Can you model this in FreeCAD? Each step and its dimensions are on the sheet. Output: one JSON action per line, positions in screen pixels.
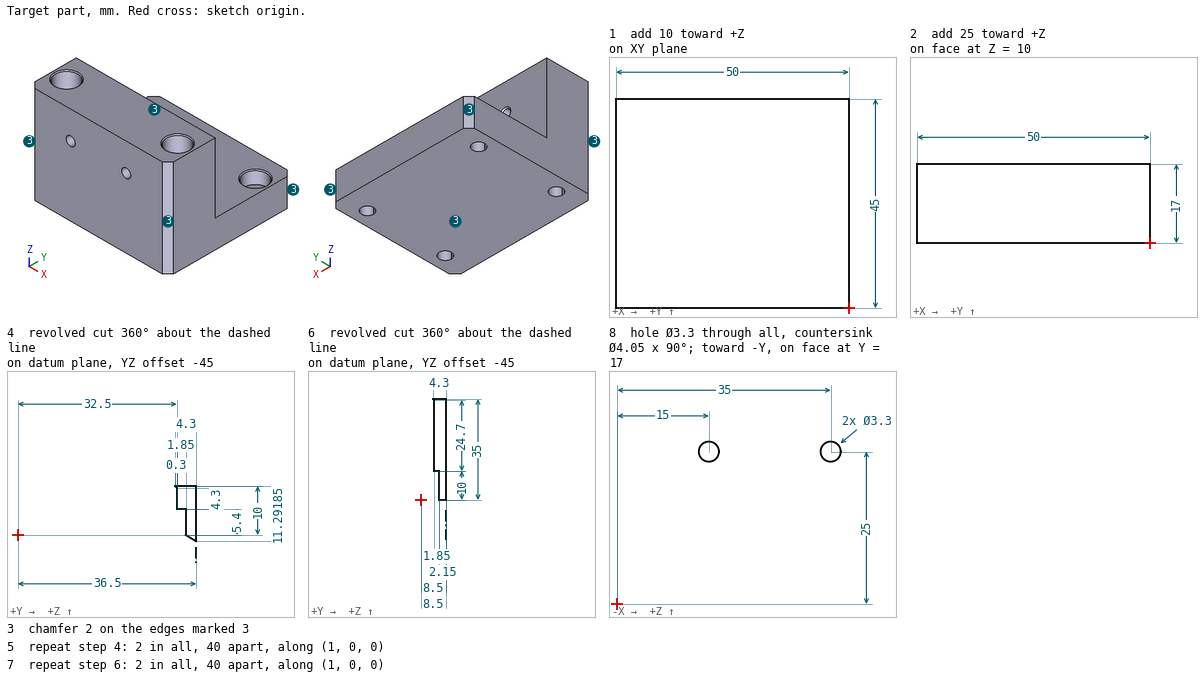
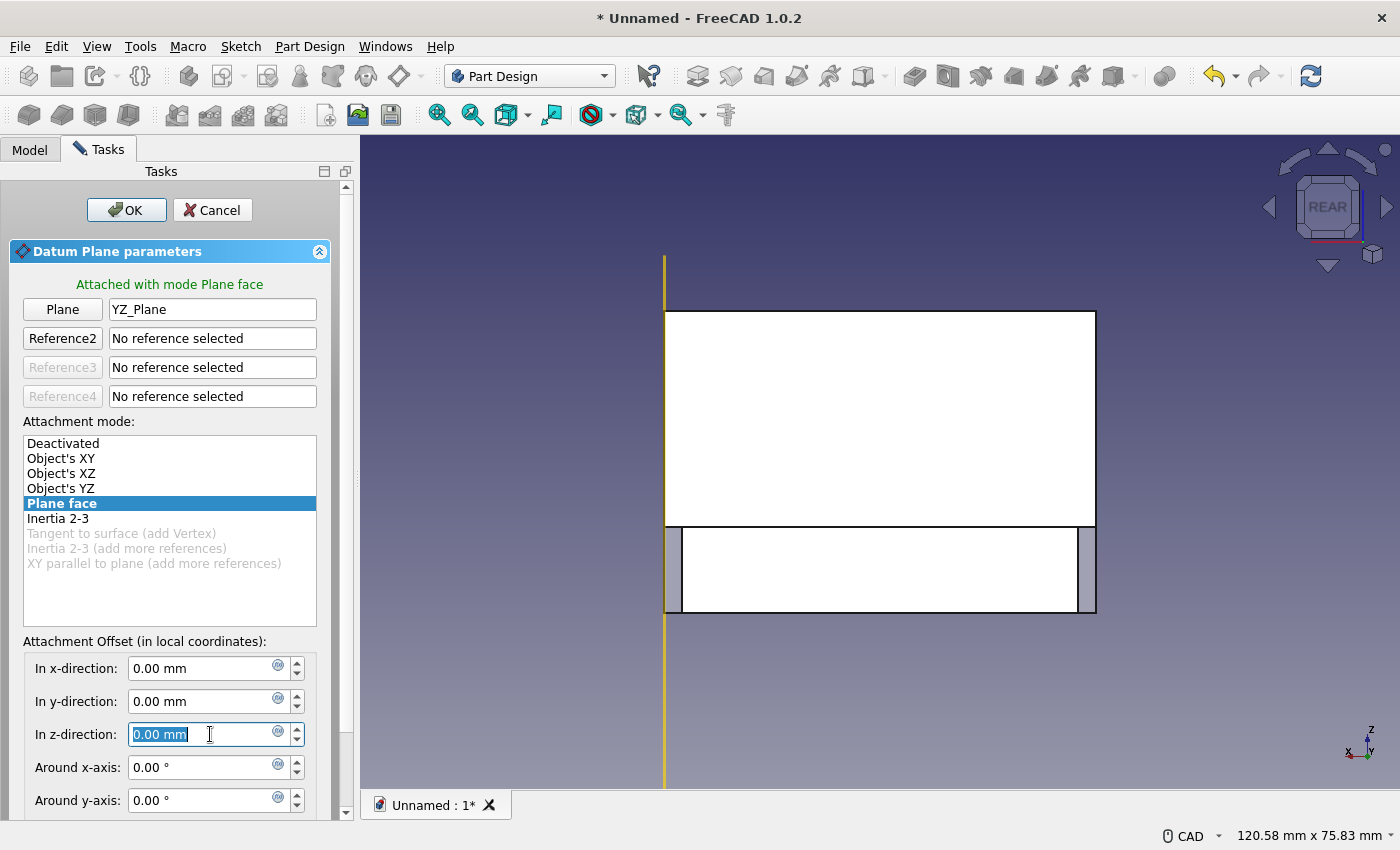
{"action": "type", "text": "-45"}
{"action": "key", "text": "Tab"}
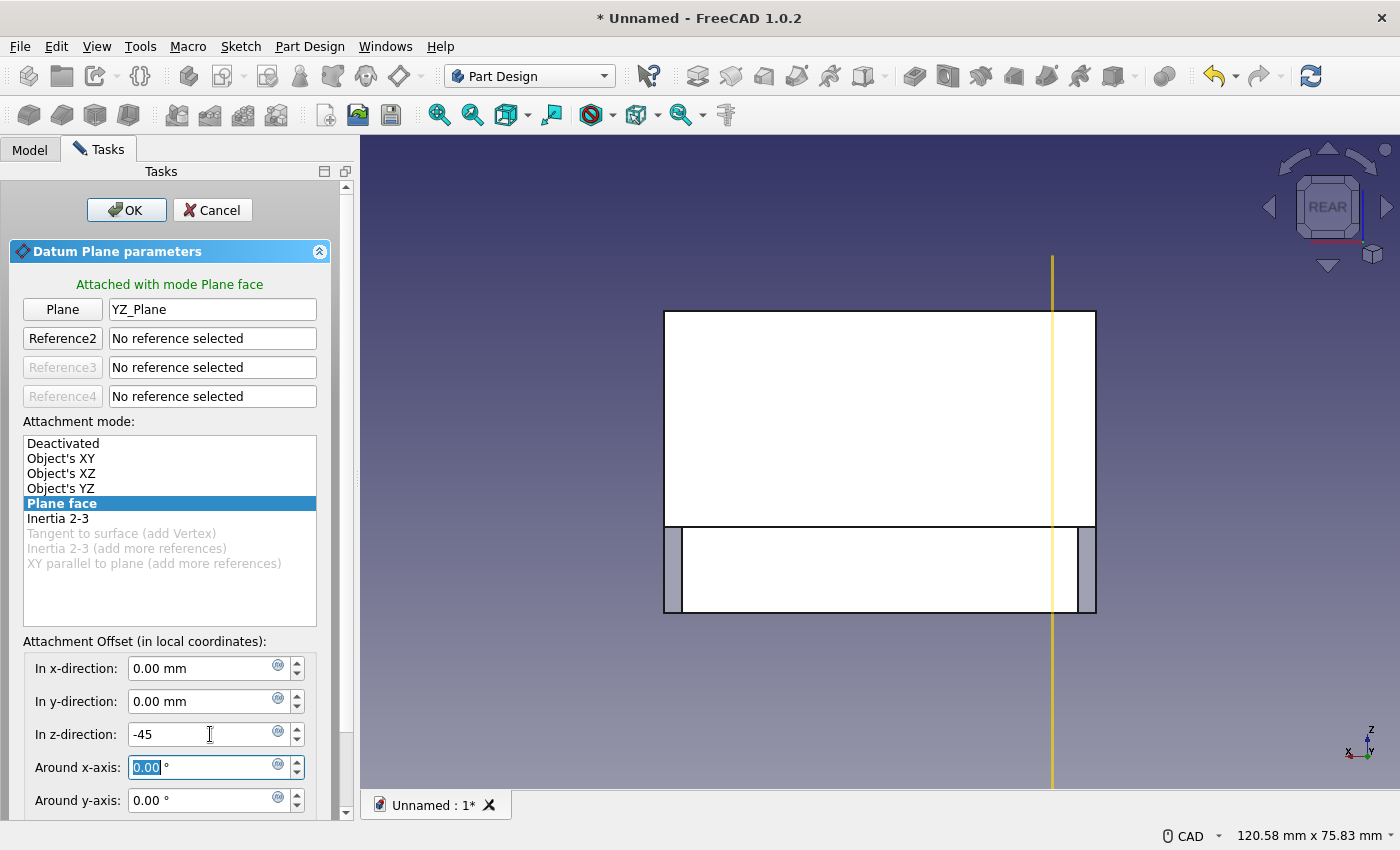
{"action": "left_click", "coordinate": [127, 210]}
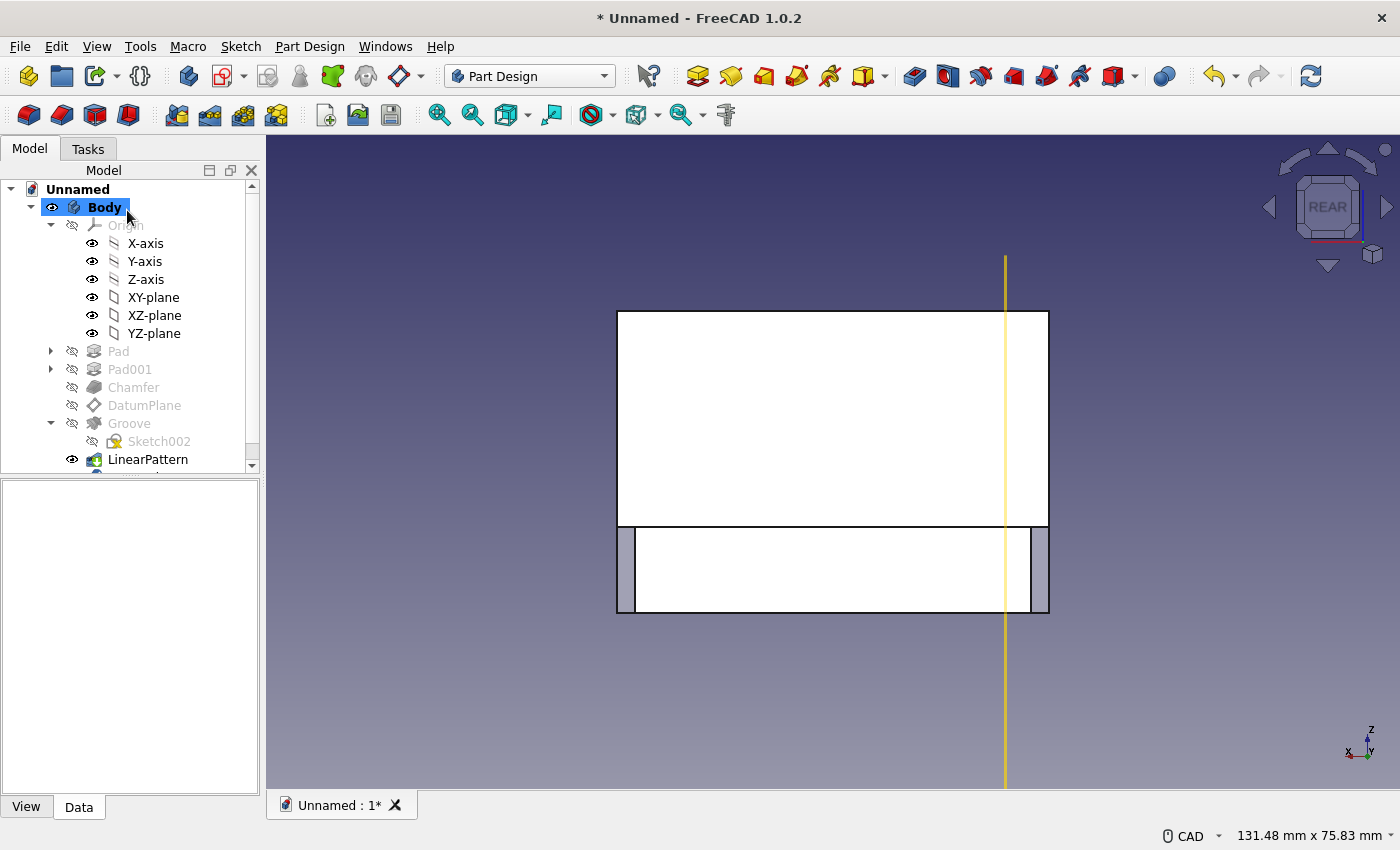
{"action": "scroll", "coordinate": [101, 329], "scroll_direction": "down", "scroll_amount": 3}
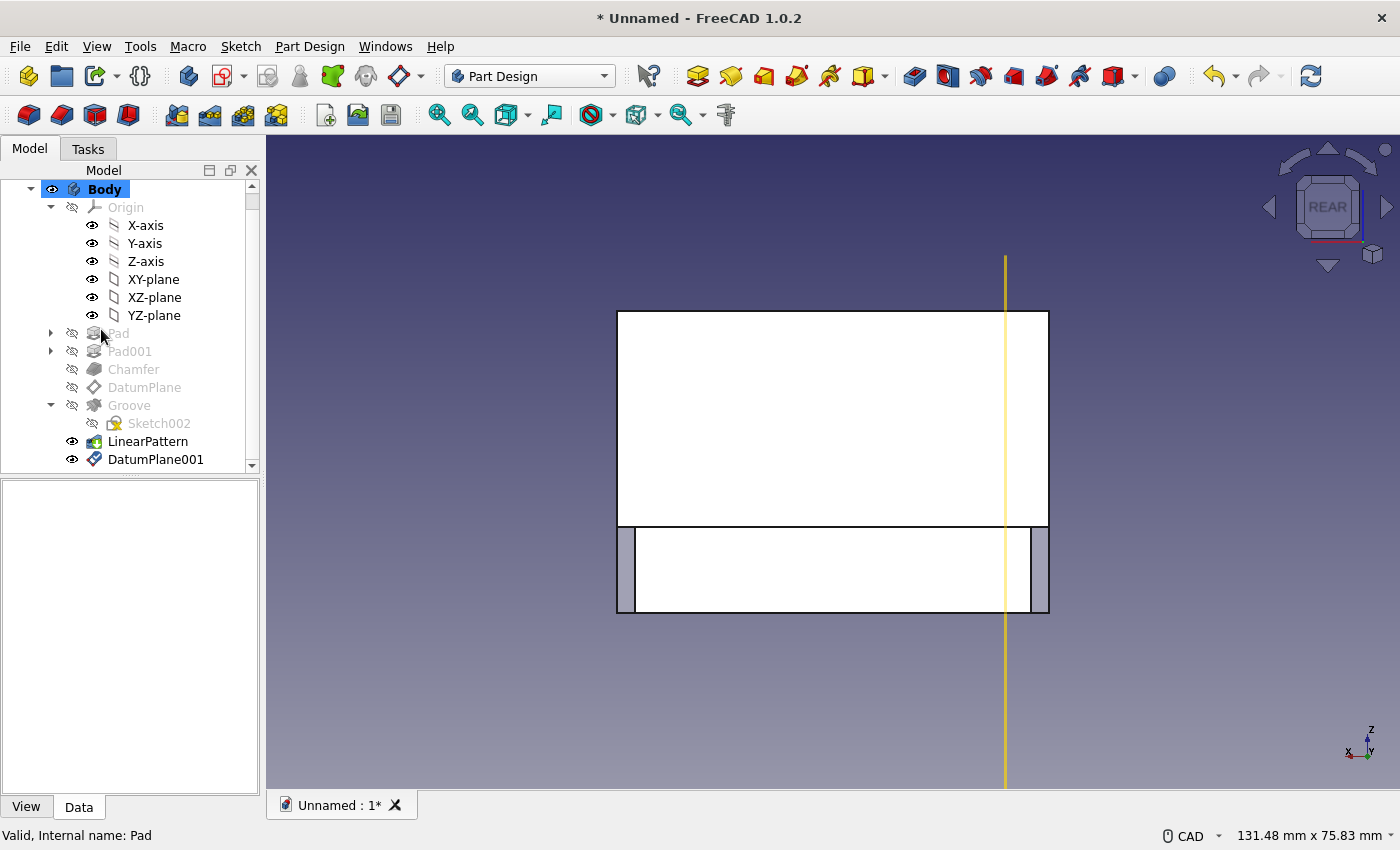
{"action": "left_click", "coordinate": [117, 459]}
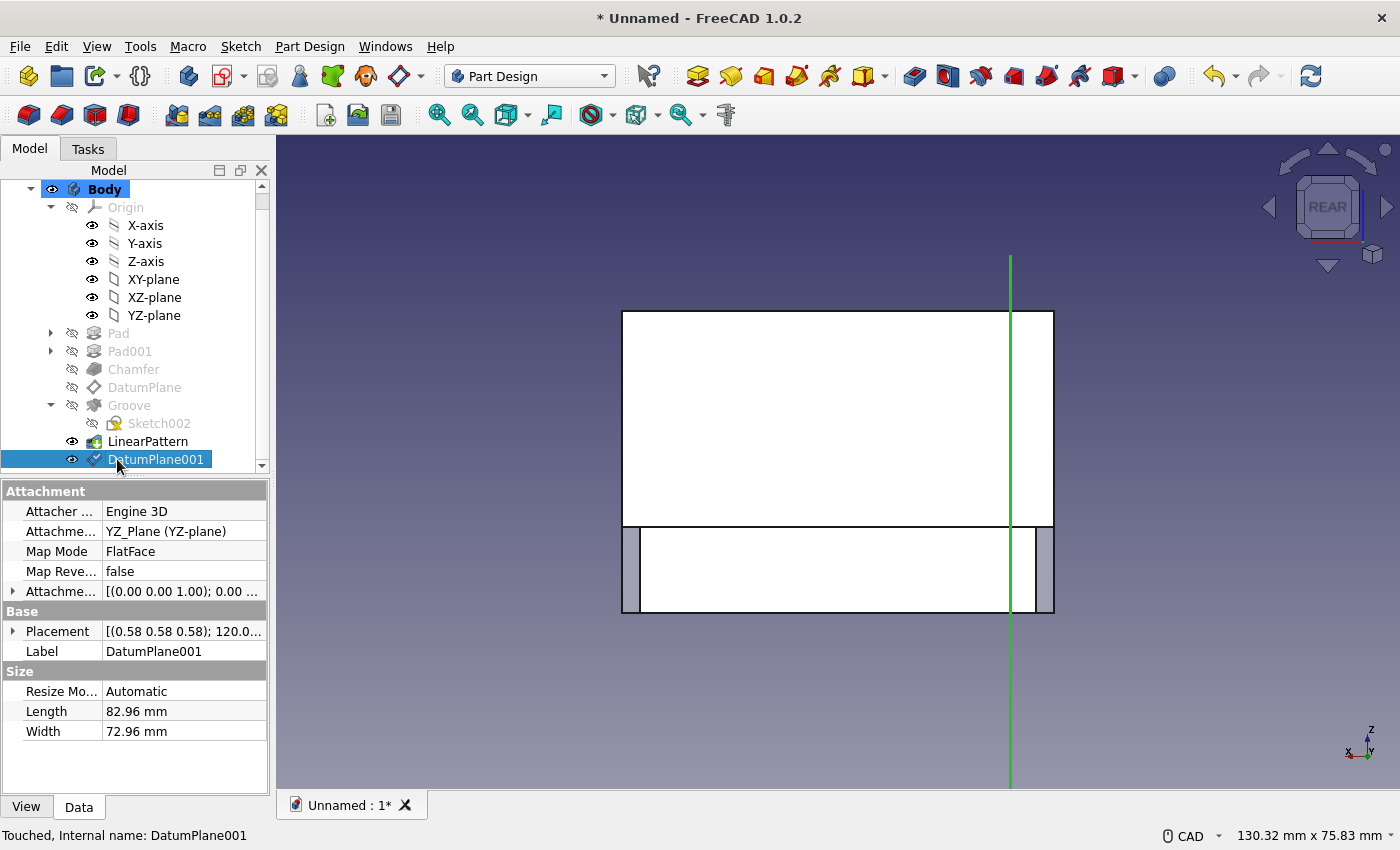
{"action": "left_click", "coordinate": [222, 76]}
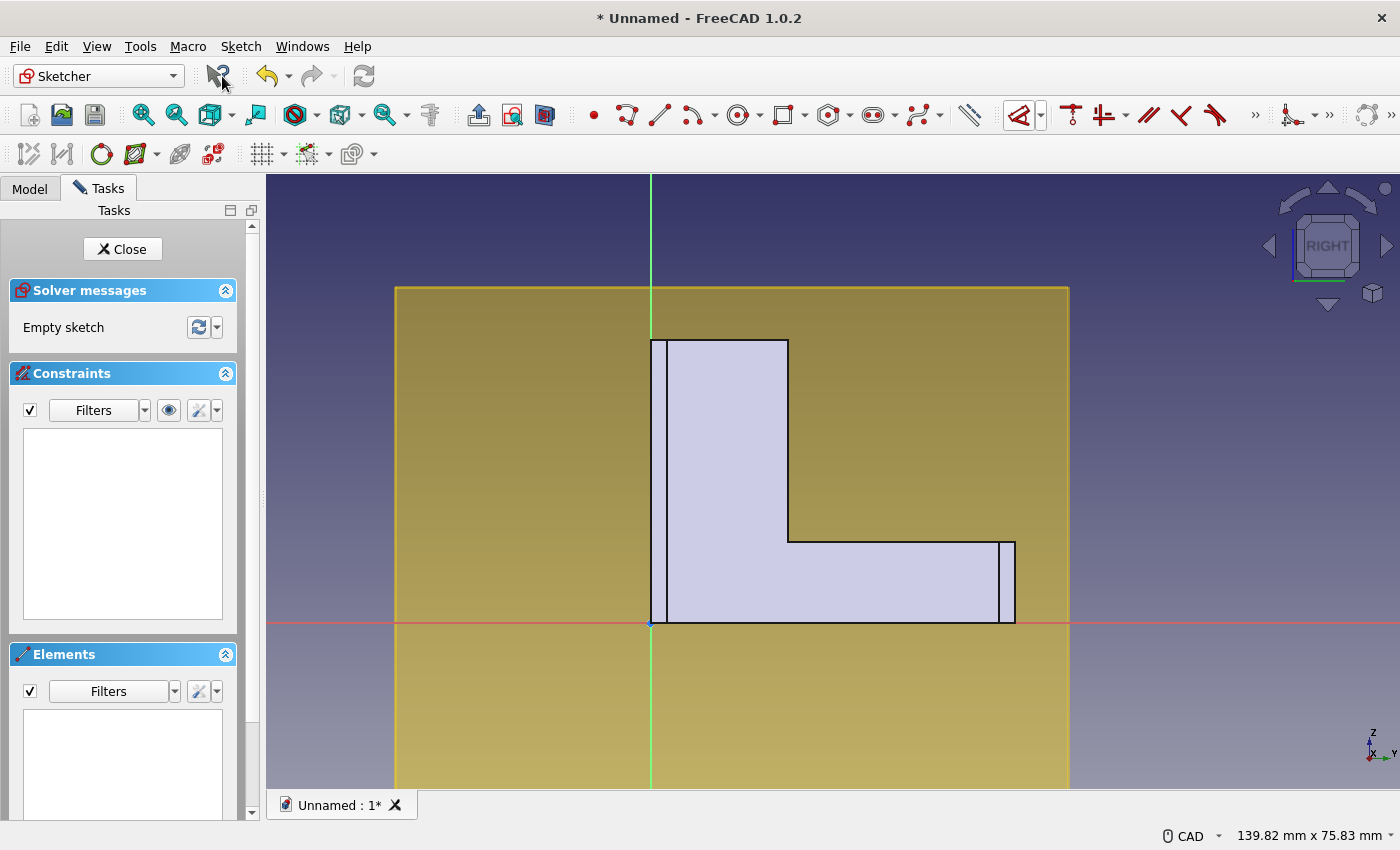
{"action": "left_click", "coordinate": [545, 116]}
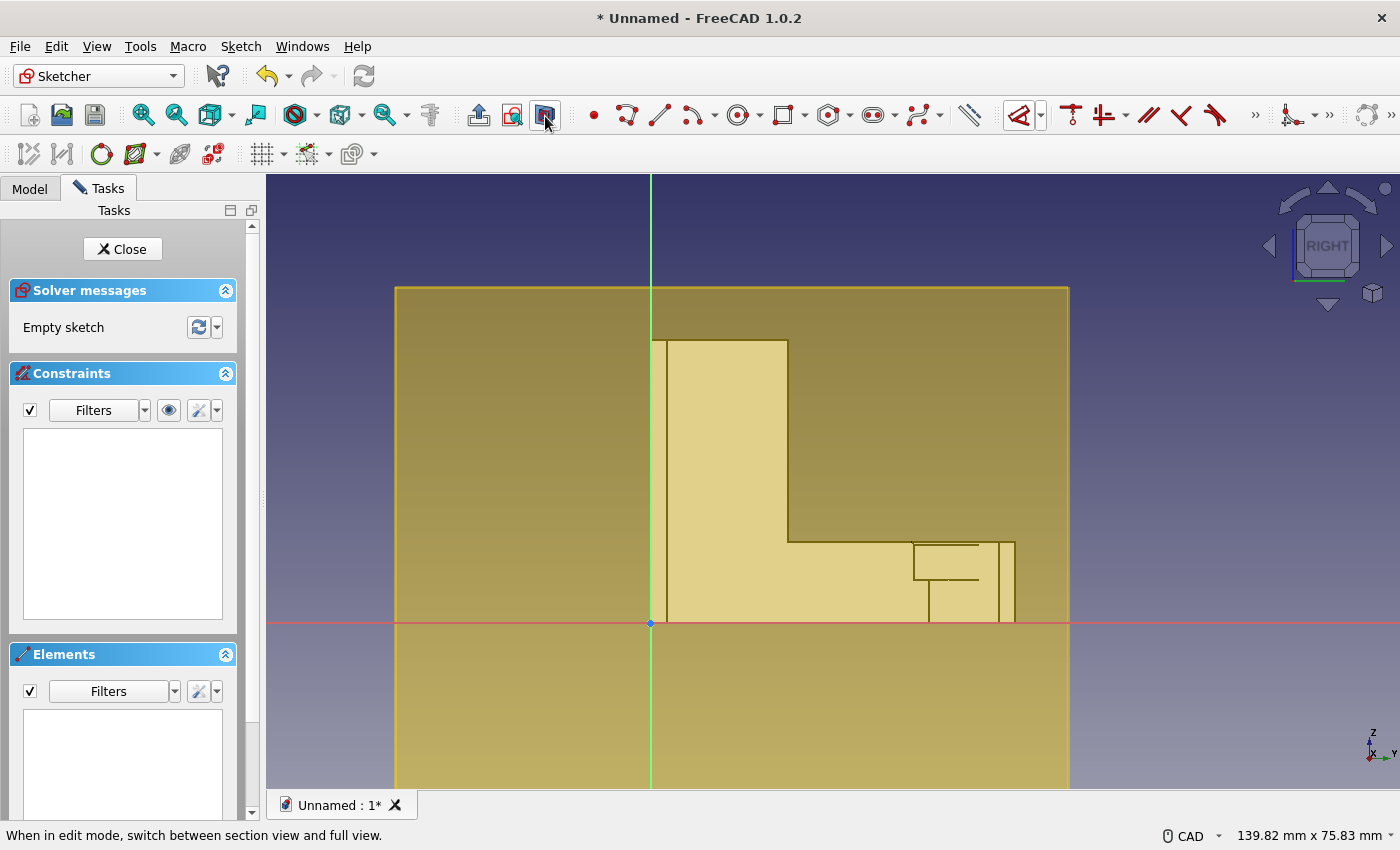
{"action": "scroll", "coordinate": [1124, 225], "scroll_direction": "down", "scroll_amount": 1}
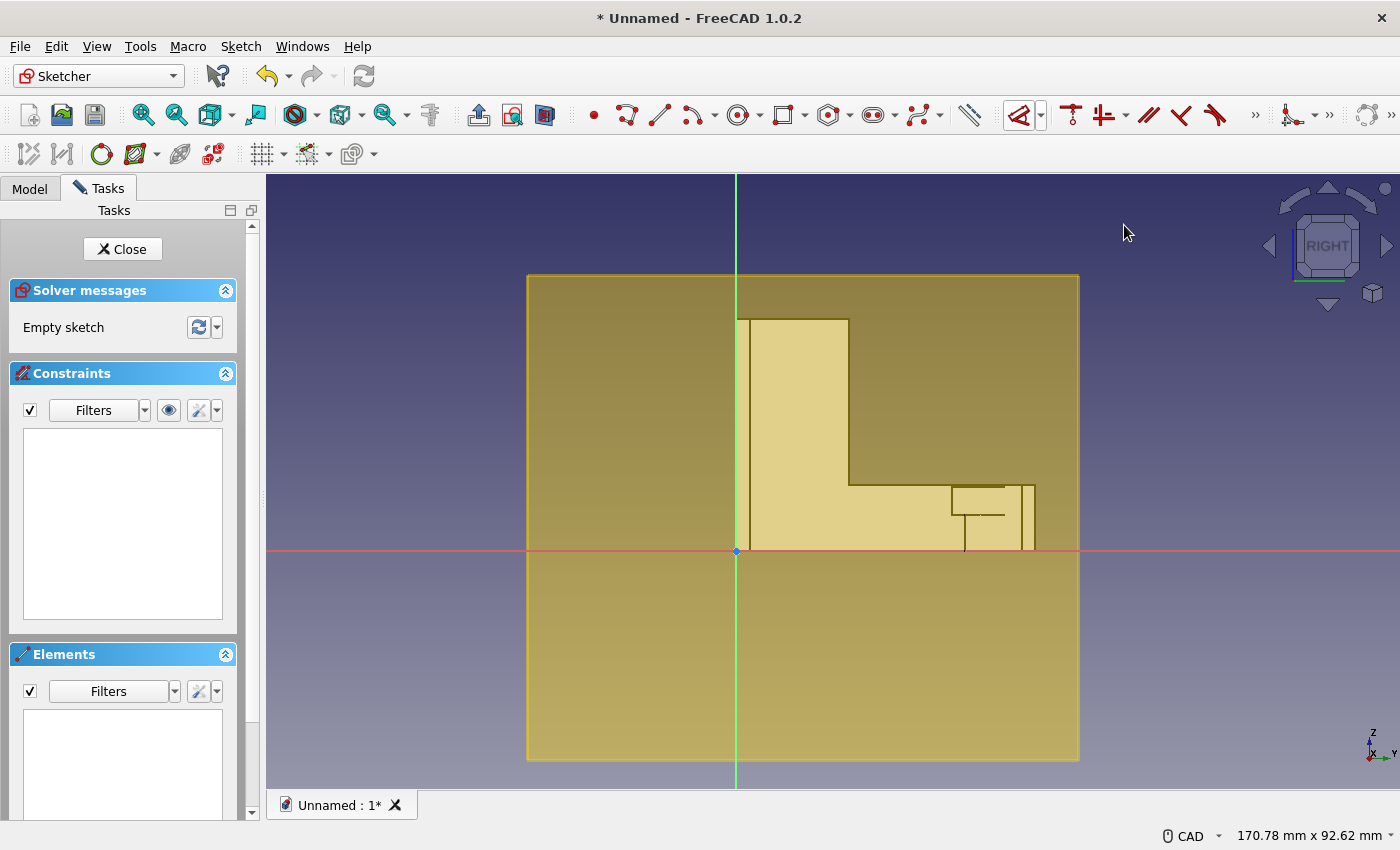
{"action": "key", "text": "g m"}